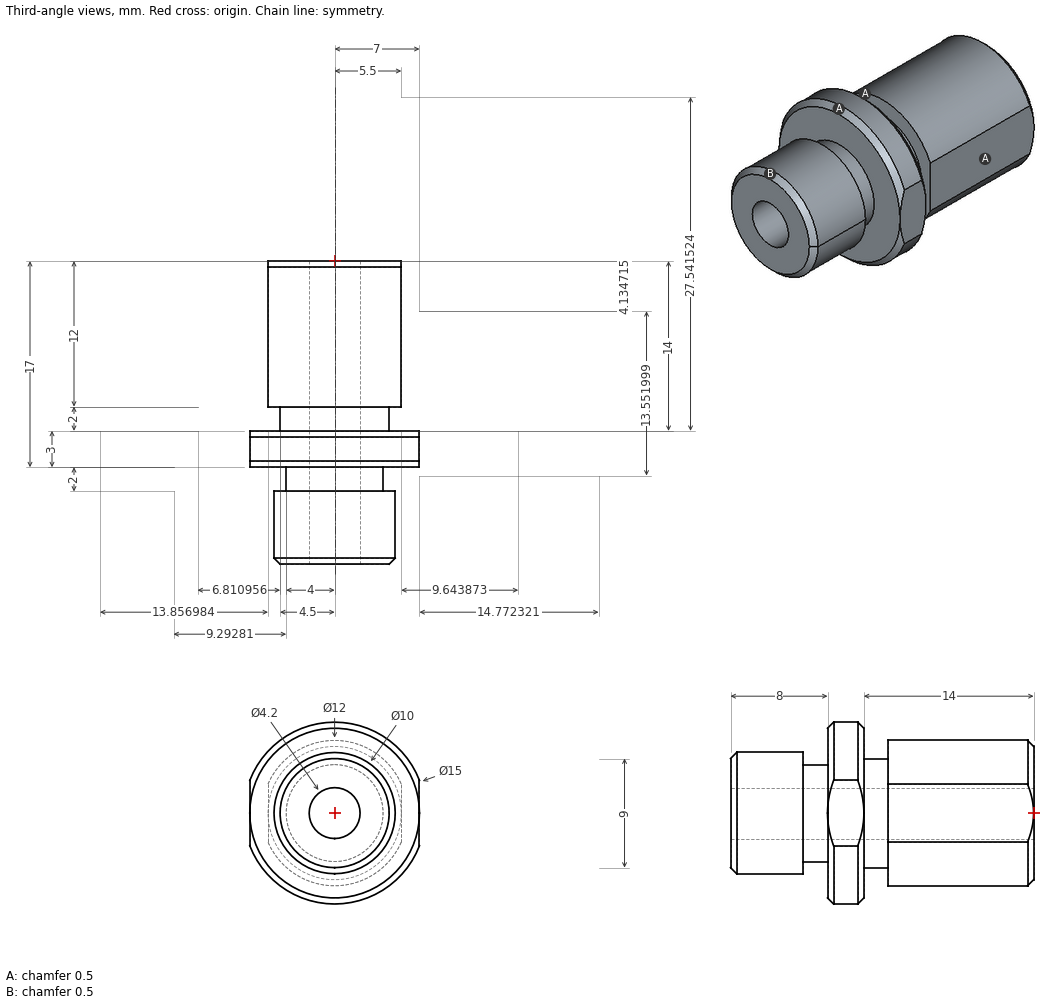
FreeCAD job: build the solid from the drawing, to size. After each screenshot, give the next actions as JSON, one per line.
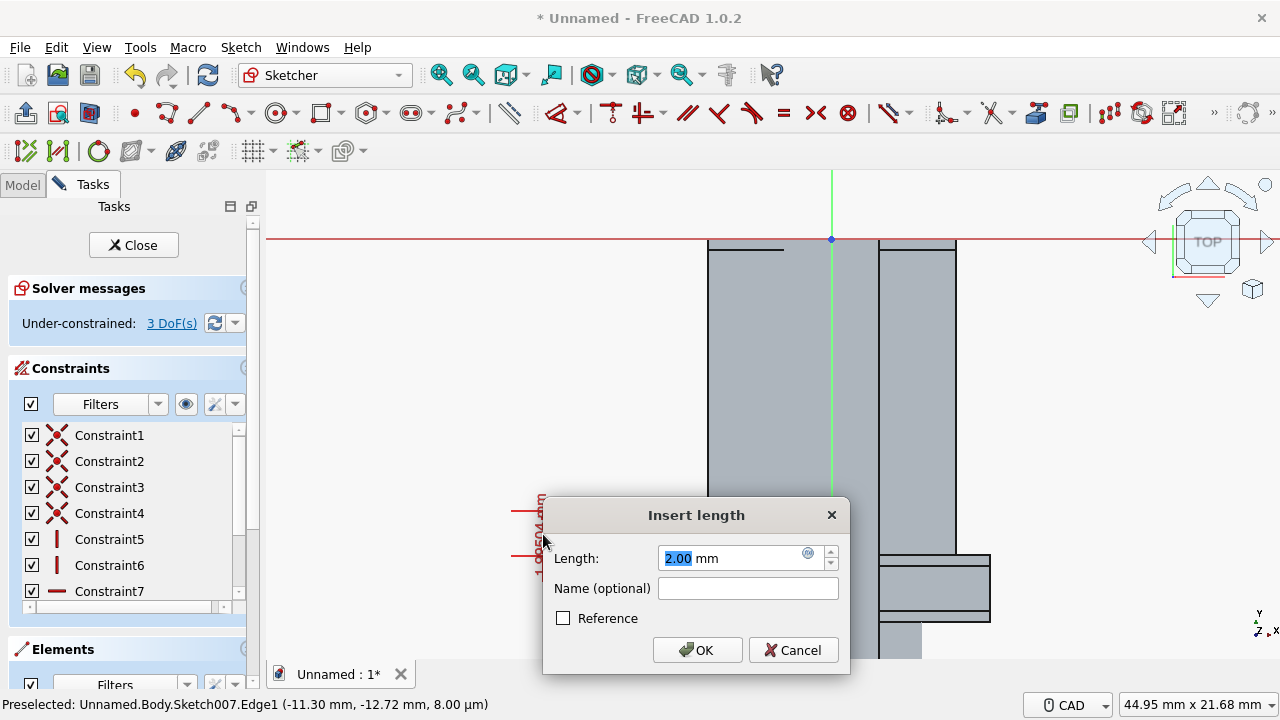
{"action": "type", "text": "2"}
{"action": "key", "text": "Return"}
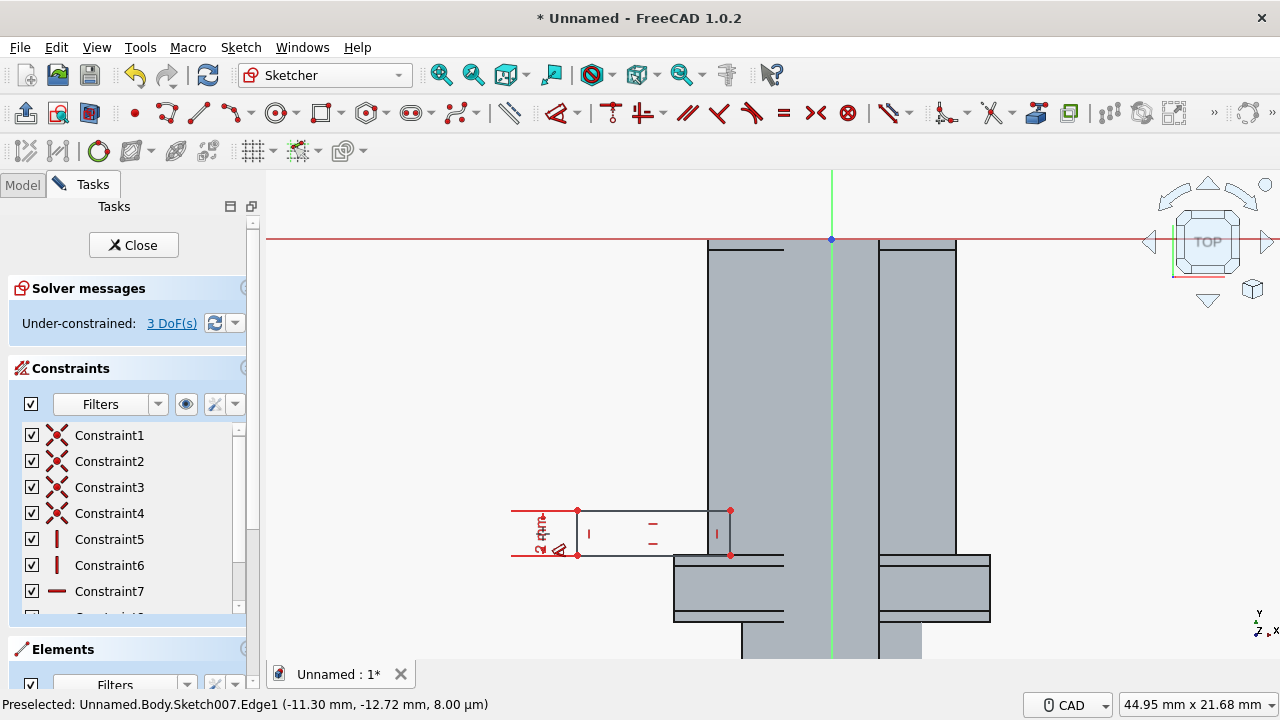
{"action": "left_click", "coordinate": [577, 511]}
{"action": "left_click", "coordinate": [866, 375]}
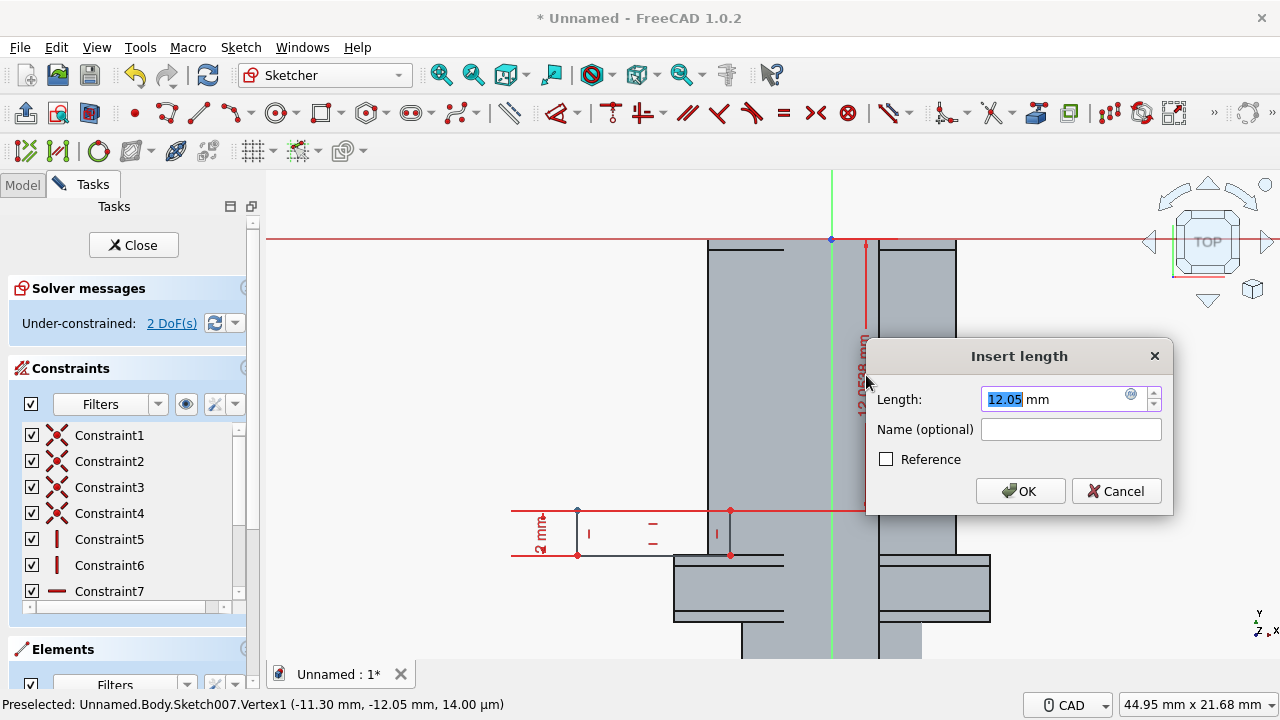
{"action": "type", "text": "12"}
{"action": "key", "text": "Return"}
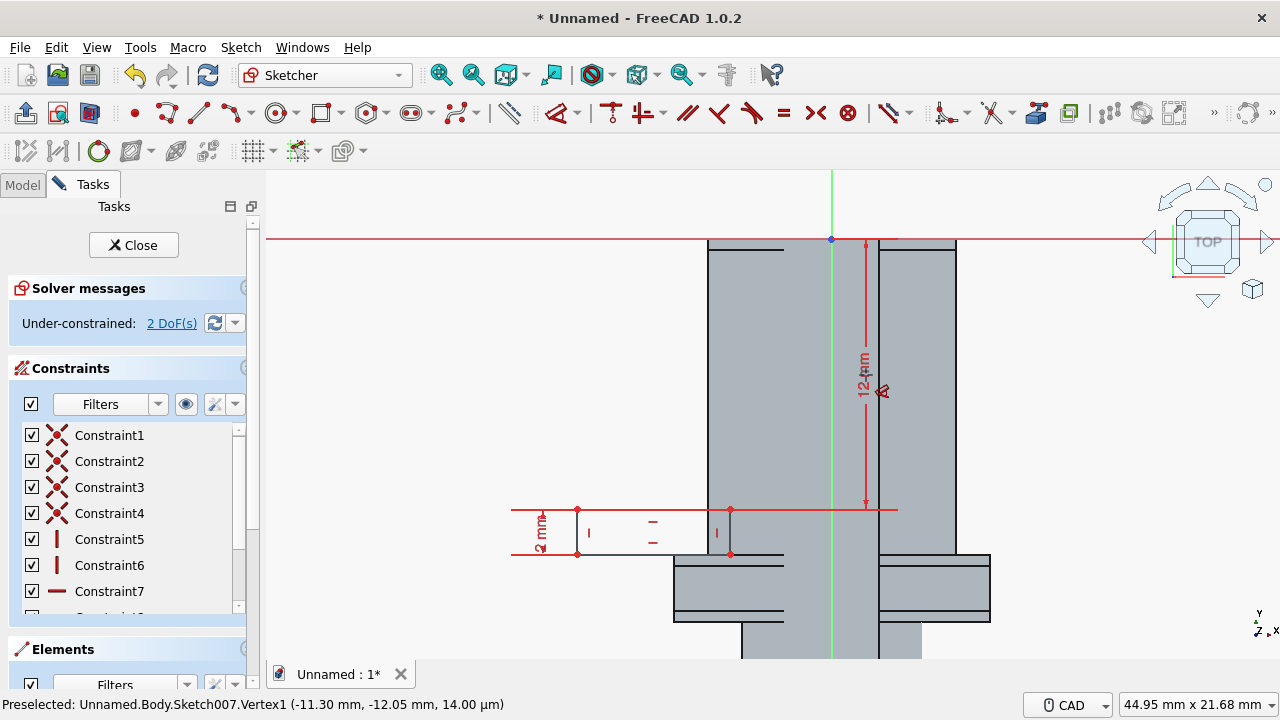
{"action": "left_click", "coordinate": [730, 555]}
{"action": "left_click", "coordinate": [781, 205]}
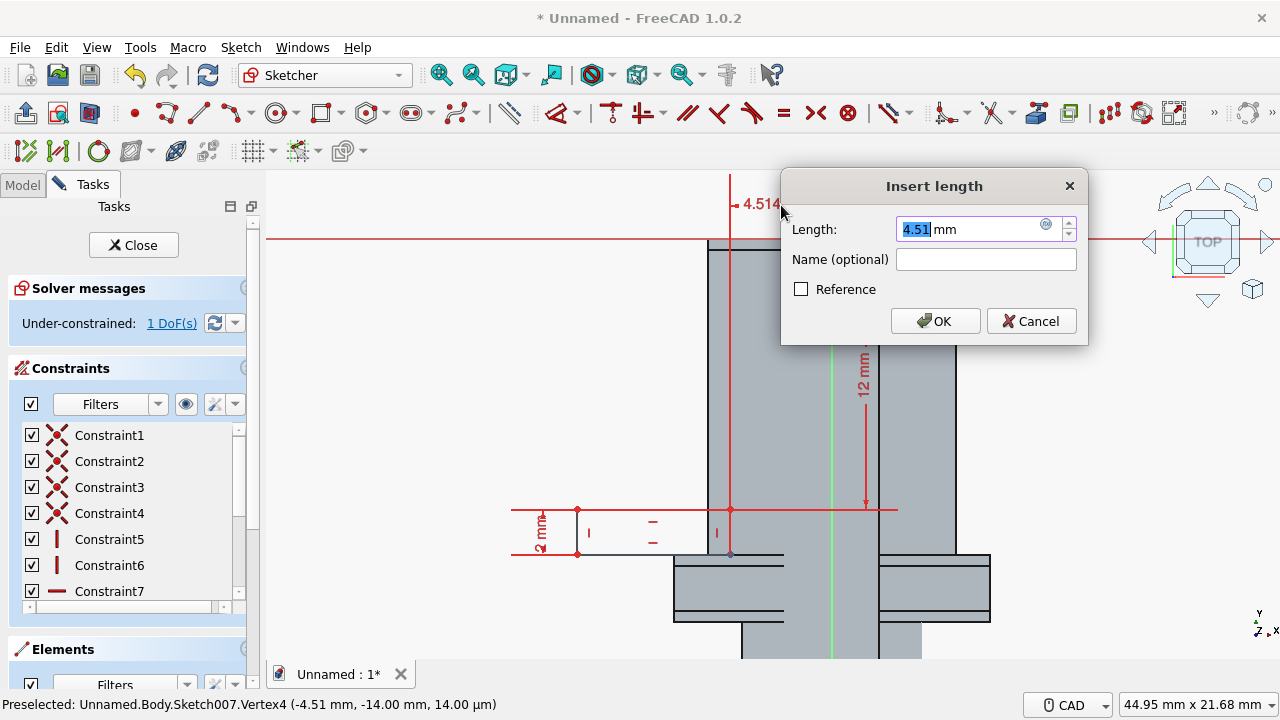
{"action": "type", "text": "4.5"}
{"action": "key", "text": "Return"}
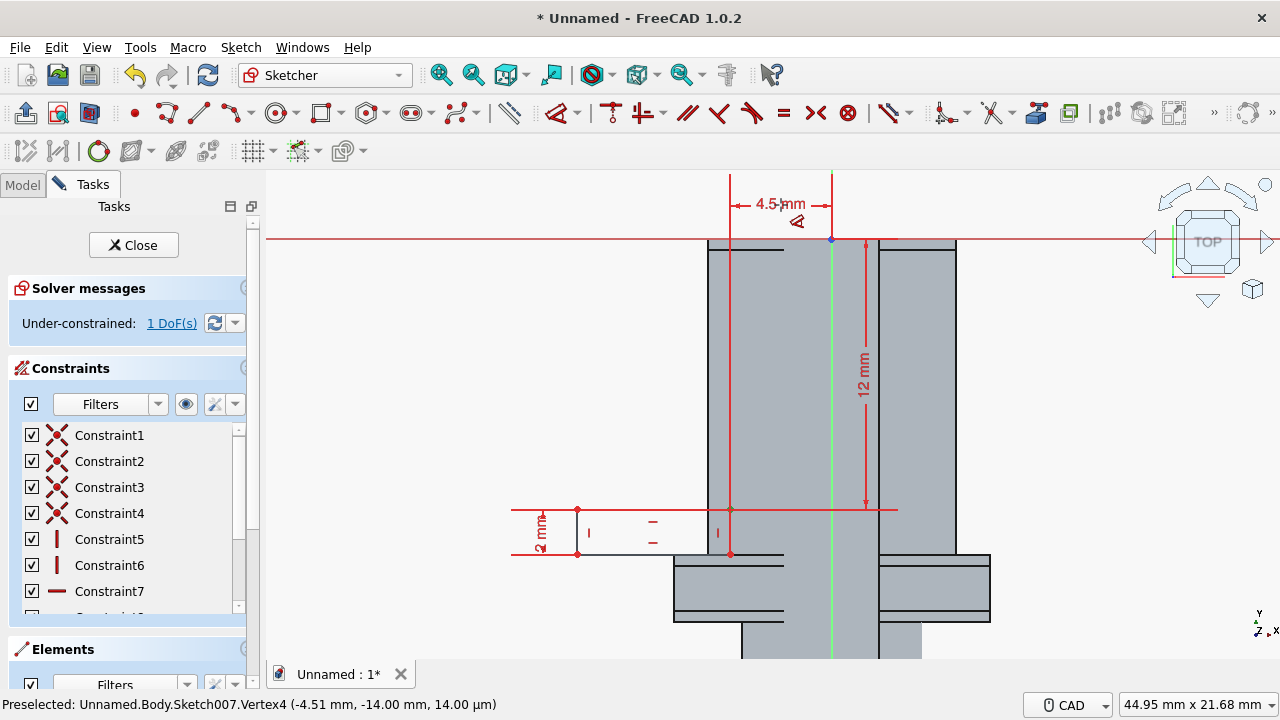
{"action": "left_click", "coordinate": [623, 555]}
{"action": "left_click", "coordinate": [654, 589]}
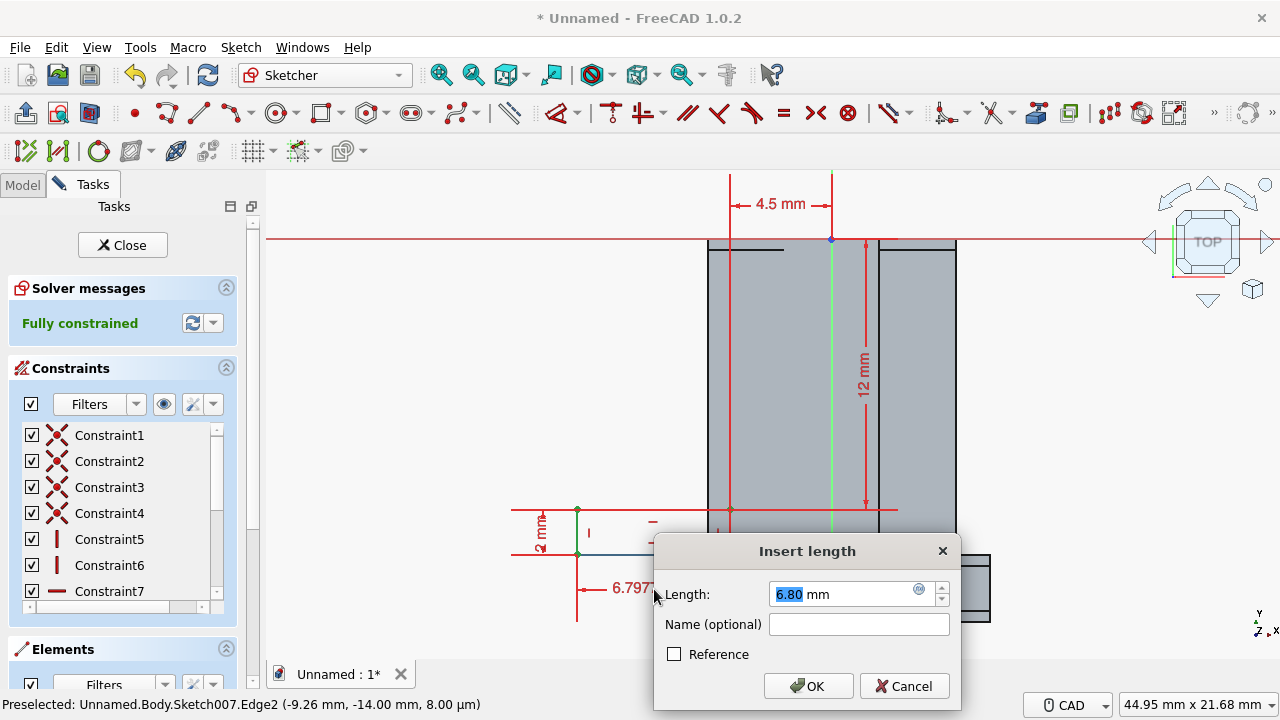
{"action": "type", "text": "6.810956"}
{"action": "key", "text": "Return"}
{"action": "key", "text": "Escape"}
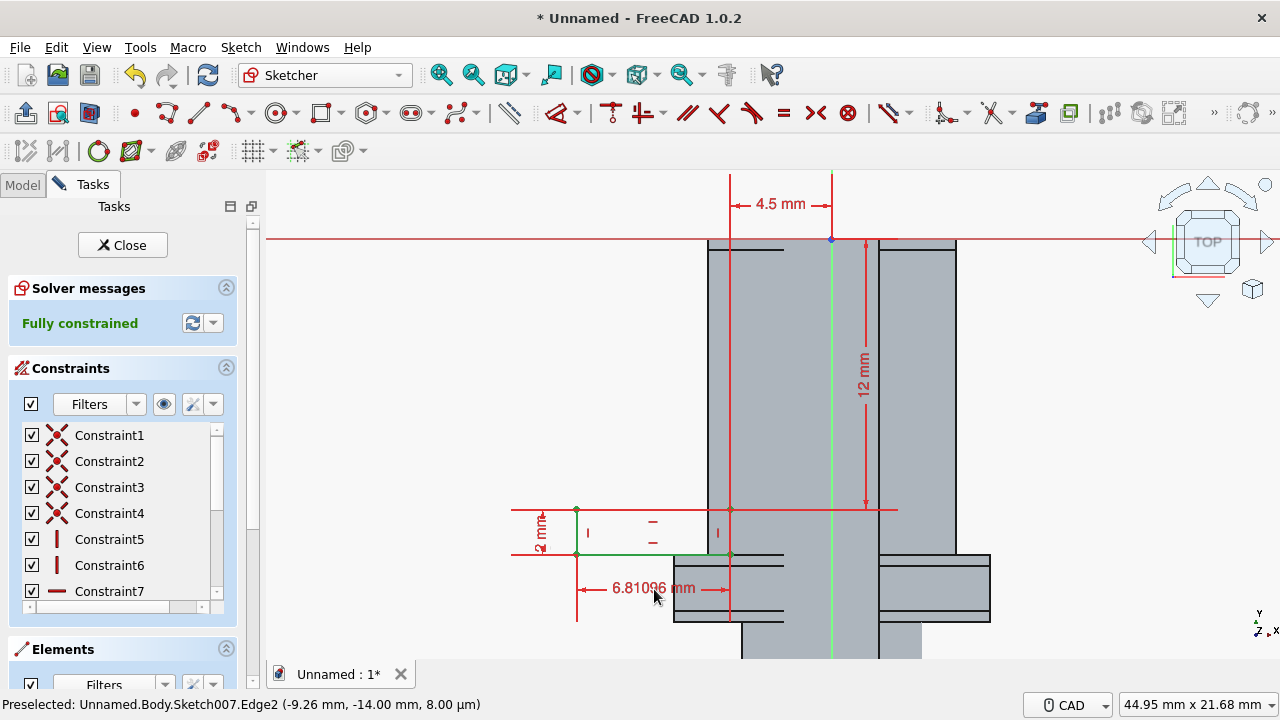
{"action": "left_click", "coordinate": [123, 245]}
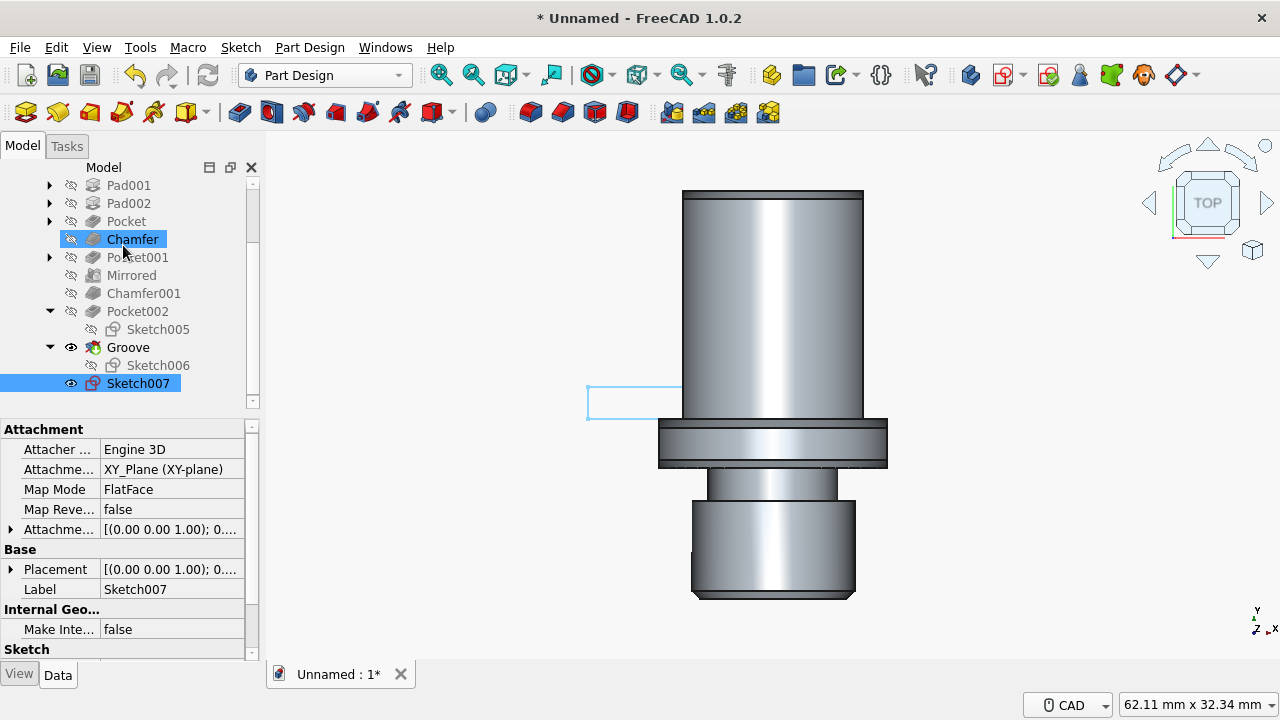
{"action": "left_click", "coordinate": [304, 112]}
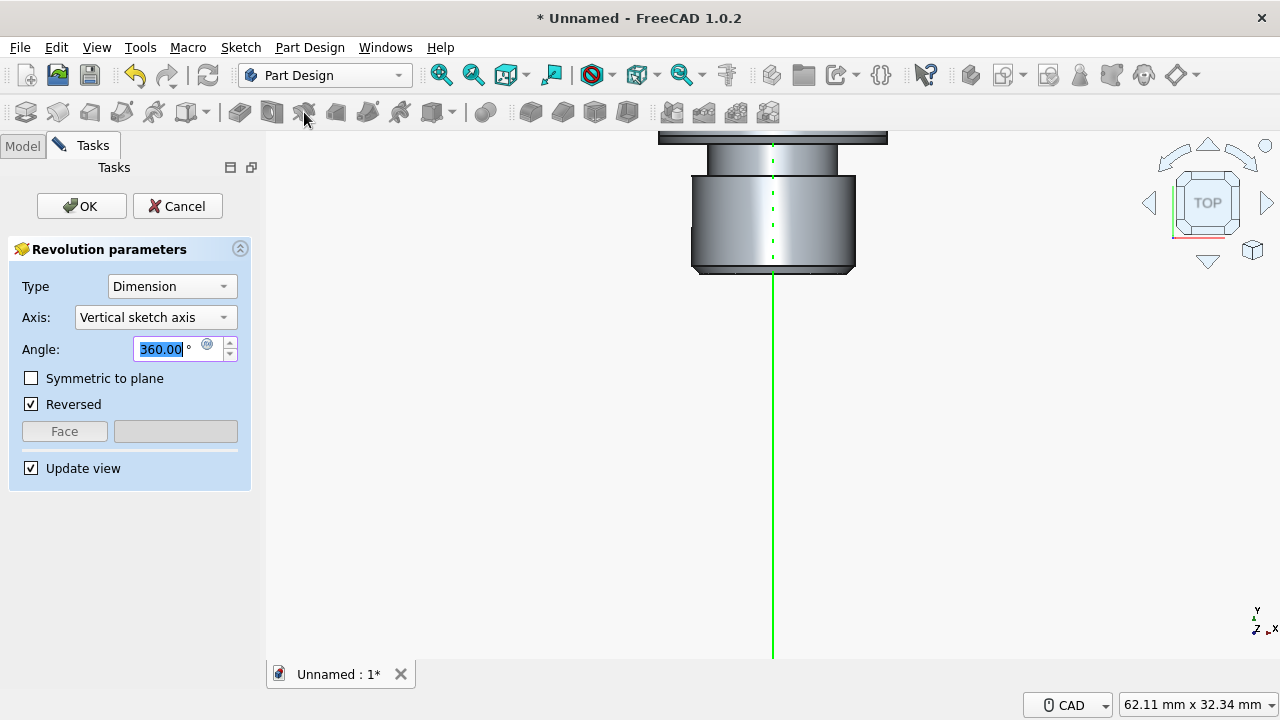
{"action": "left_click", "coordinate": [82, 206]}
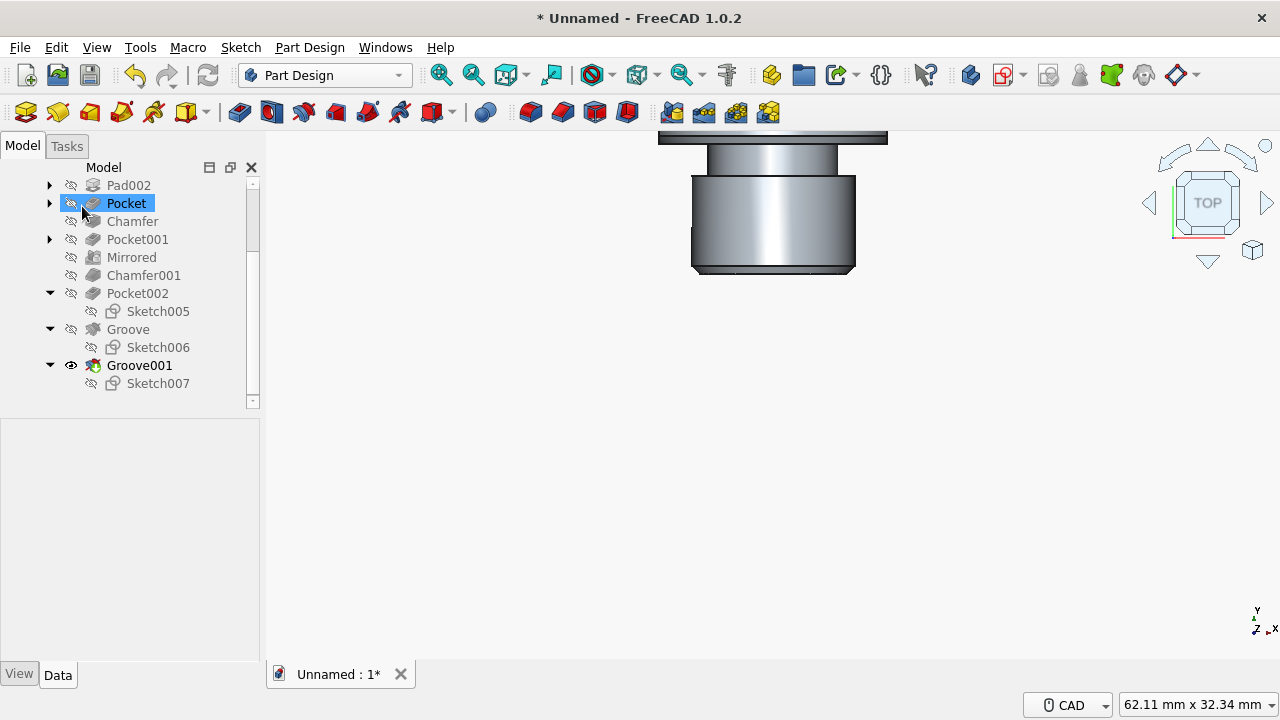
{"action": "key", "text": "0"}